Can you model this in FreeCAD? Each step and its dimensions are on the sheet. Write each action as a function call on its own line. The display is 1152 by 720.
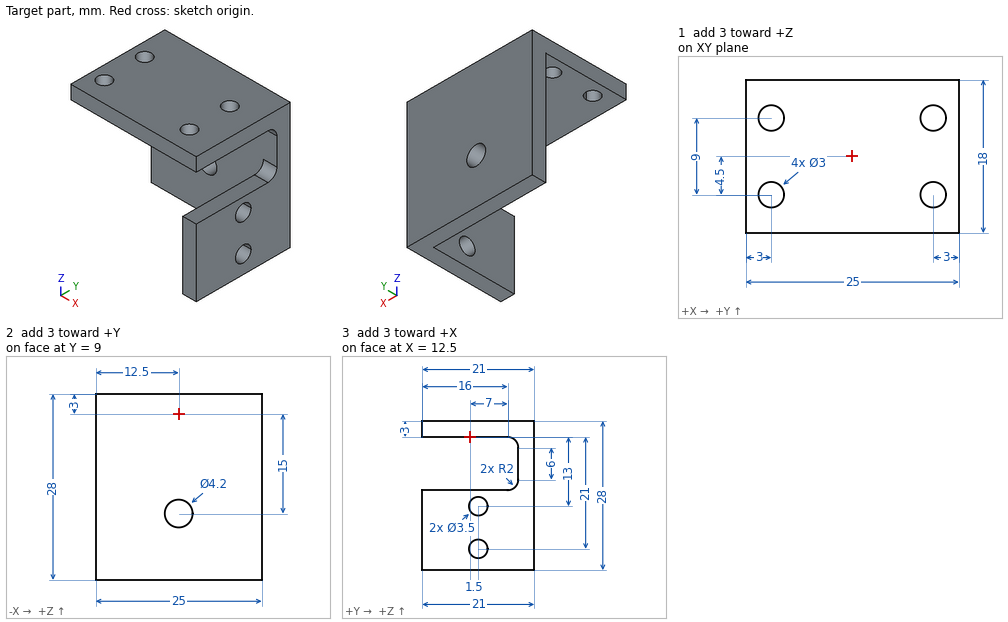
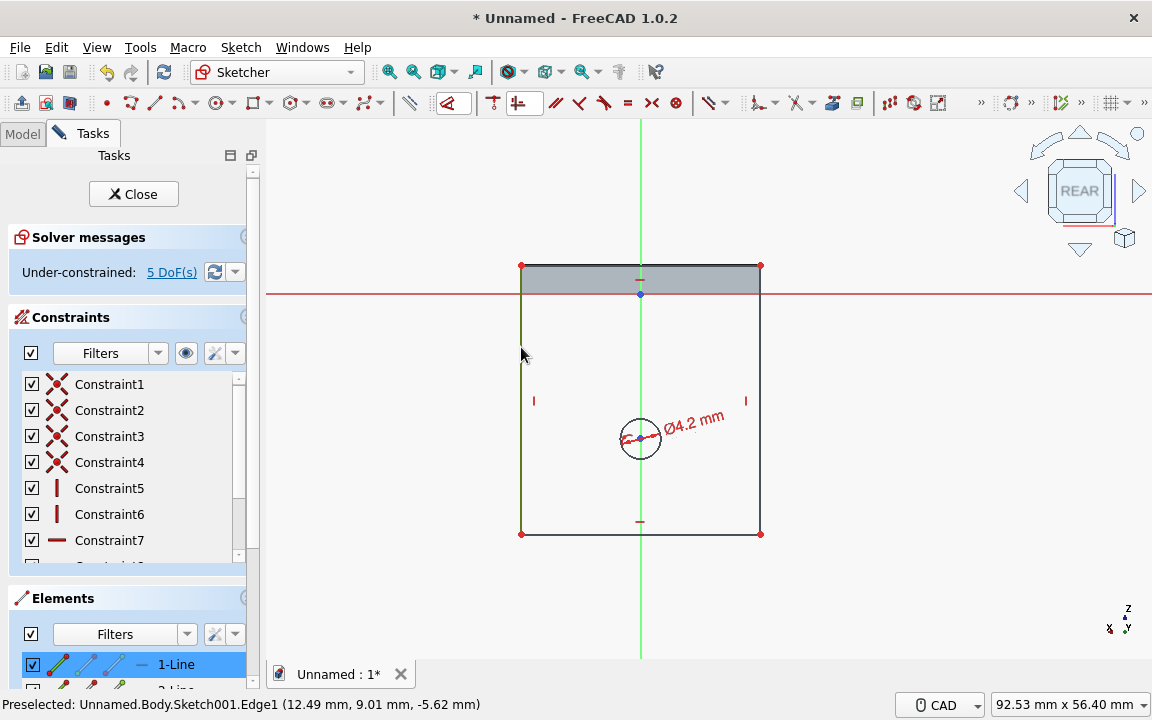
key(i)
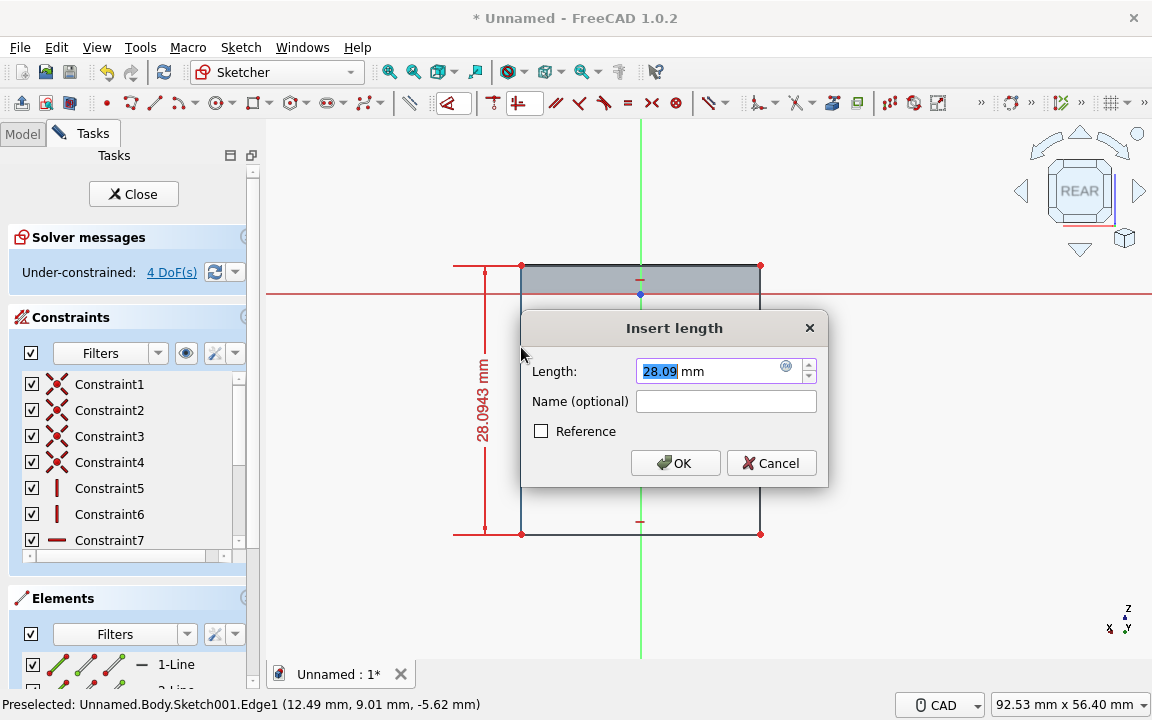
text(28)
key(Return)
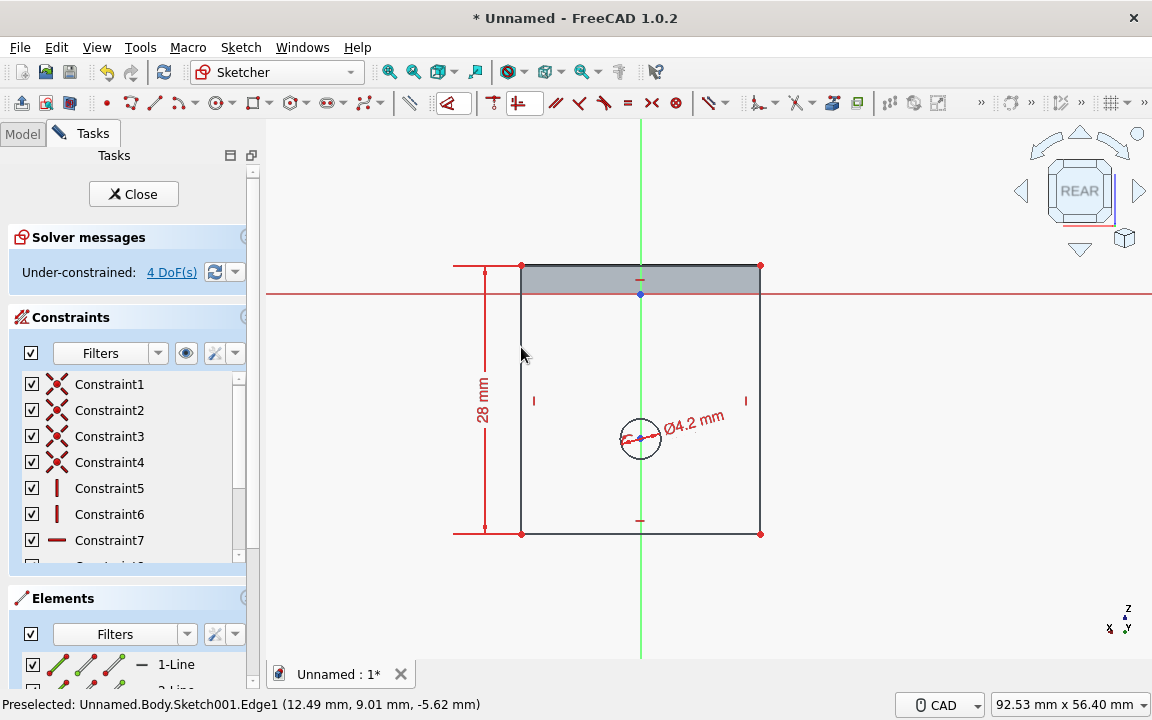
click(593, 534)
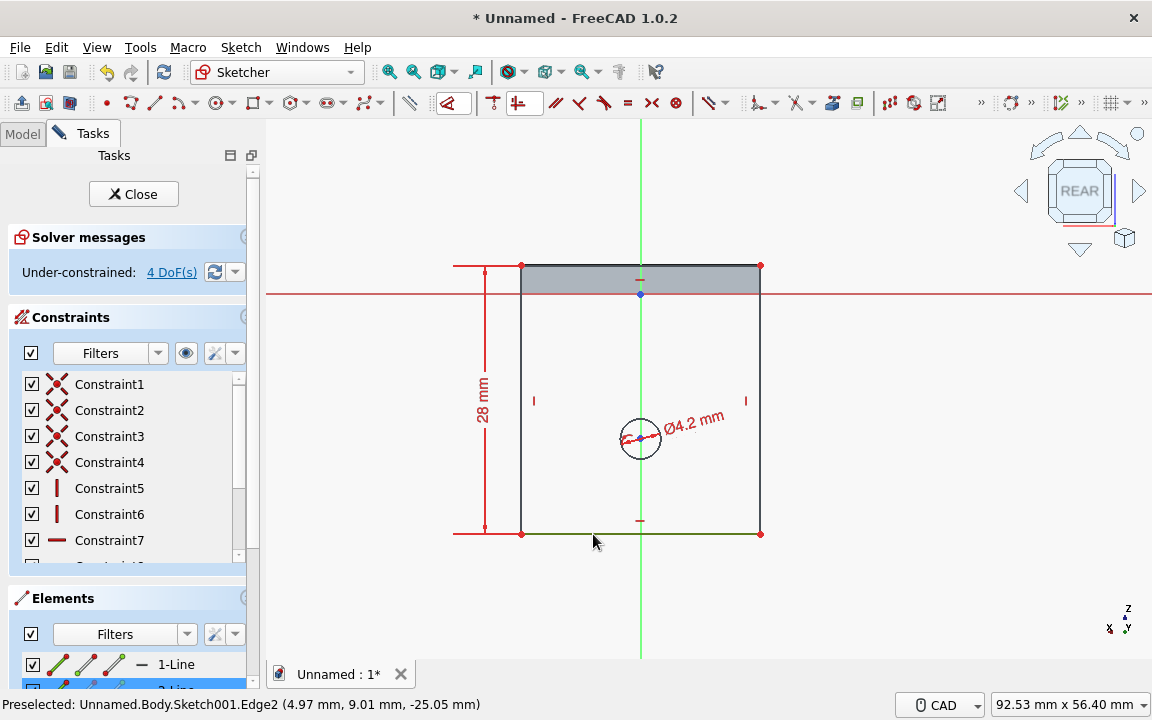
key(l)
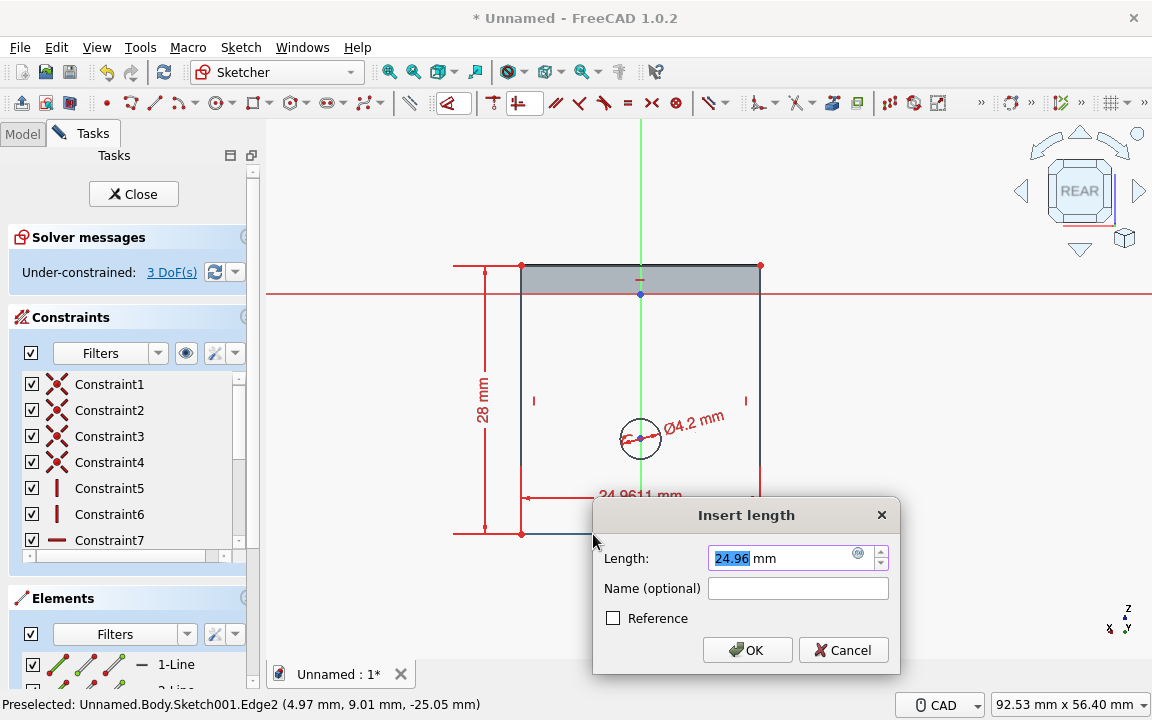
text(25)
key(Return)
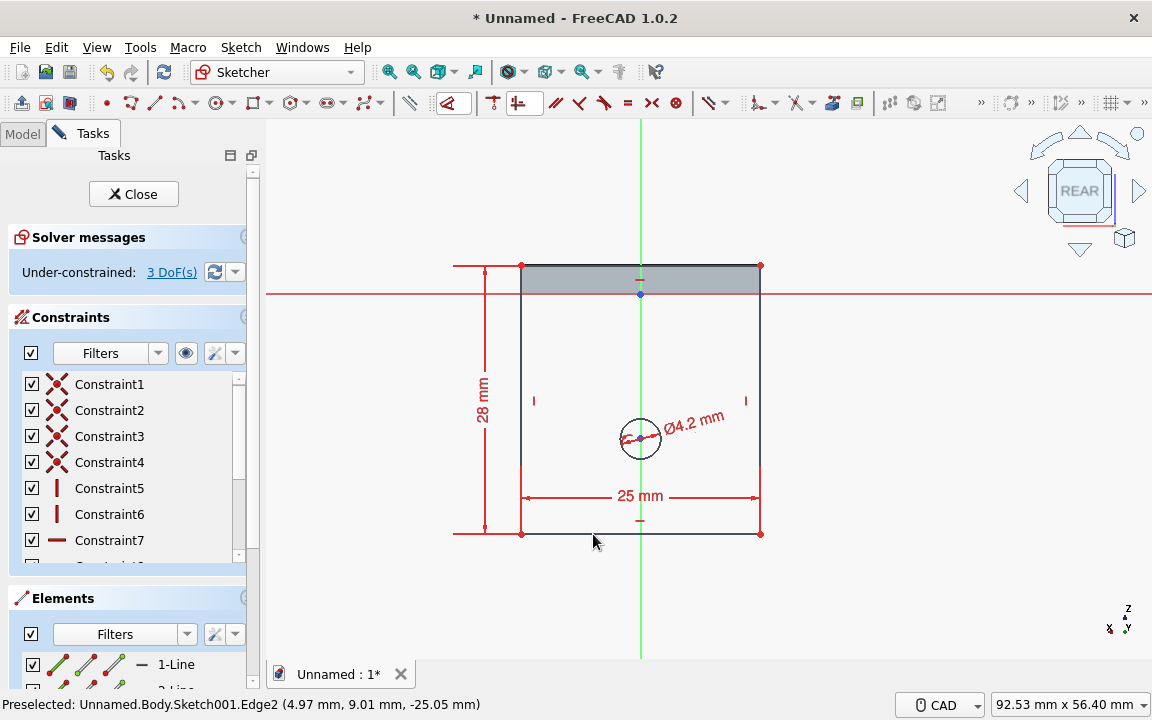
scroll(521, 266, up, 2)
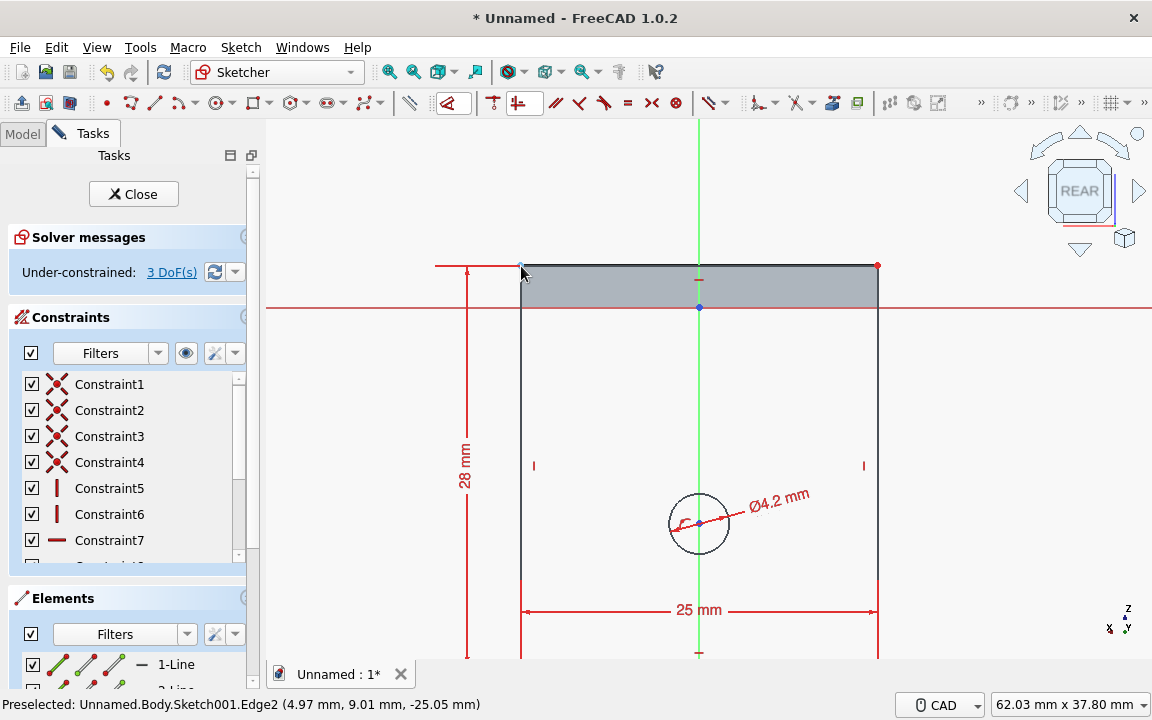
click(521, 266)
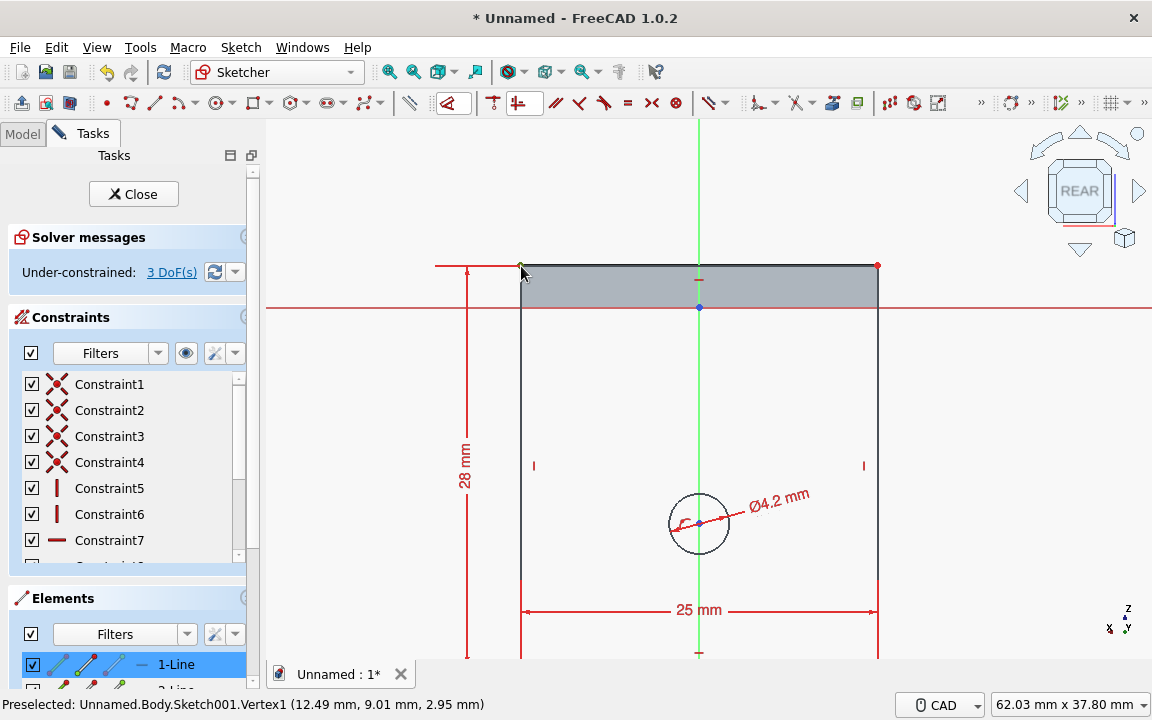
key(i)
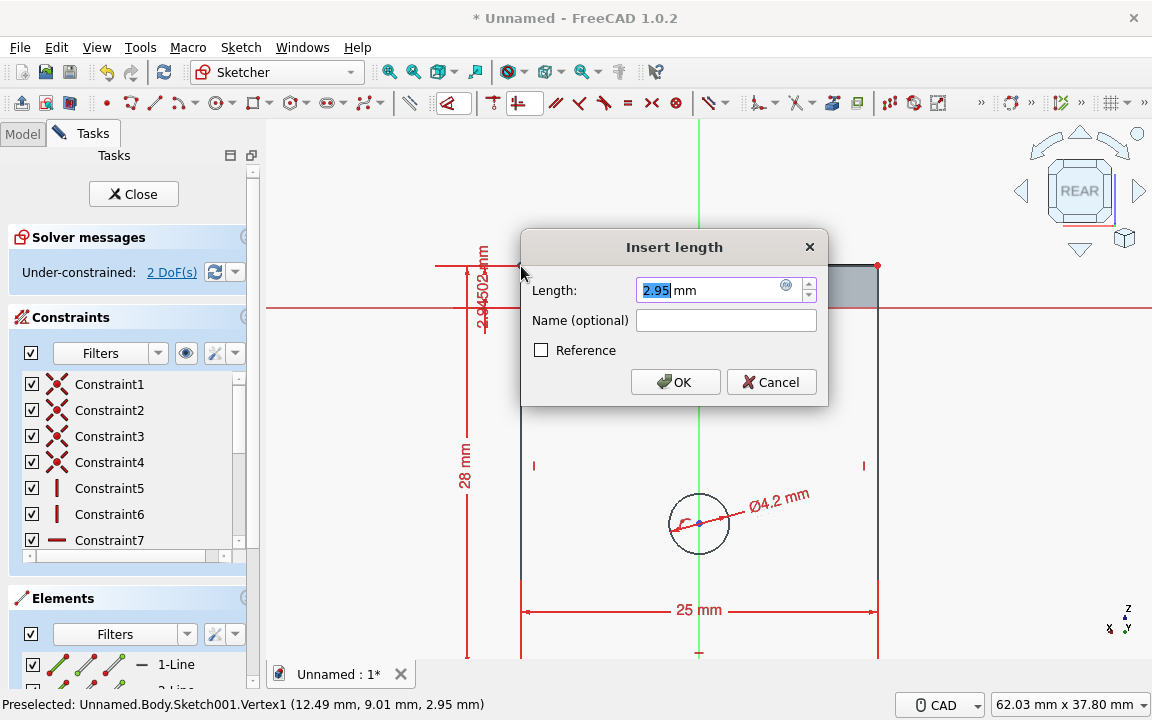
text(3)
key(Return)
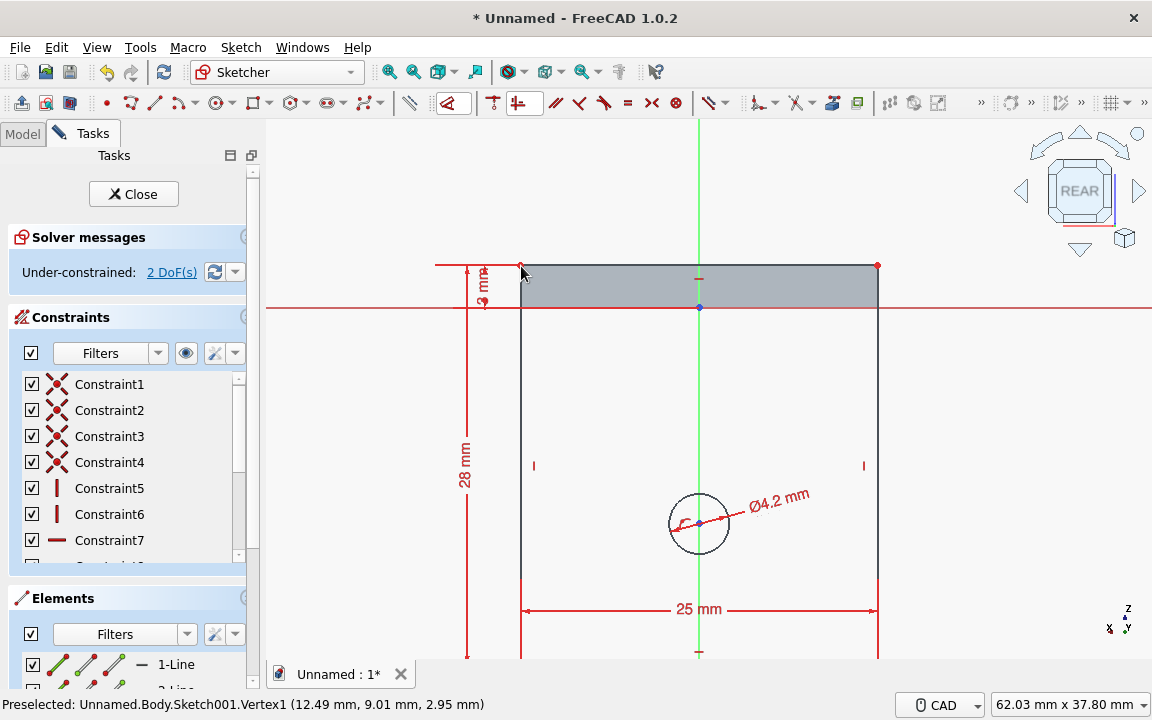
click(699, 524)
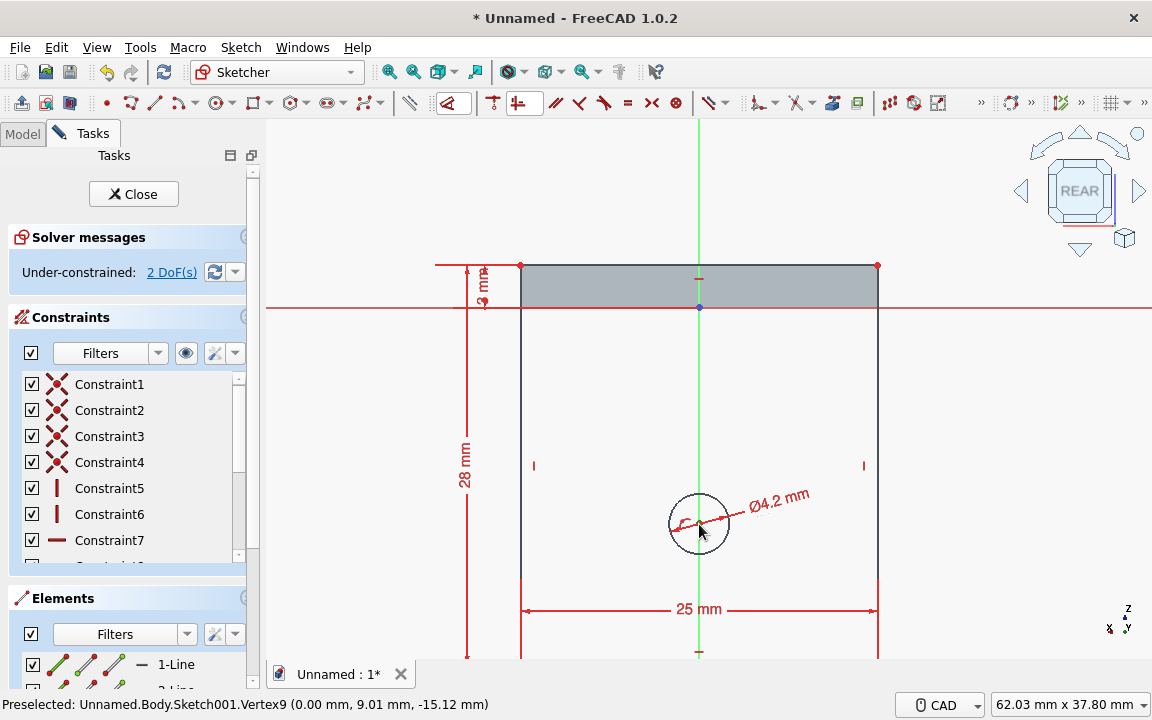
key(i)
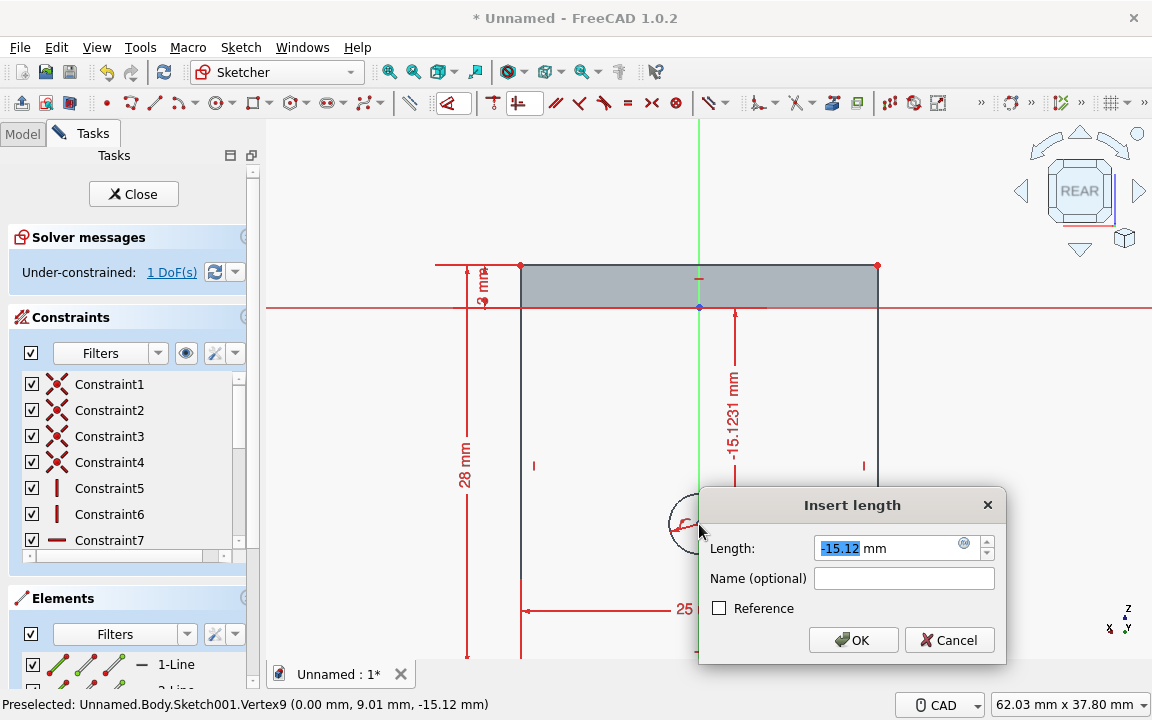
text(-15)
key(Return)